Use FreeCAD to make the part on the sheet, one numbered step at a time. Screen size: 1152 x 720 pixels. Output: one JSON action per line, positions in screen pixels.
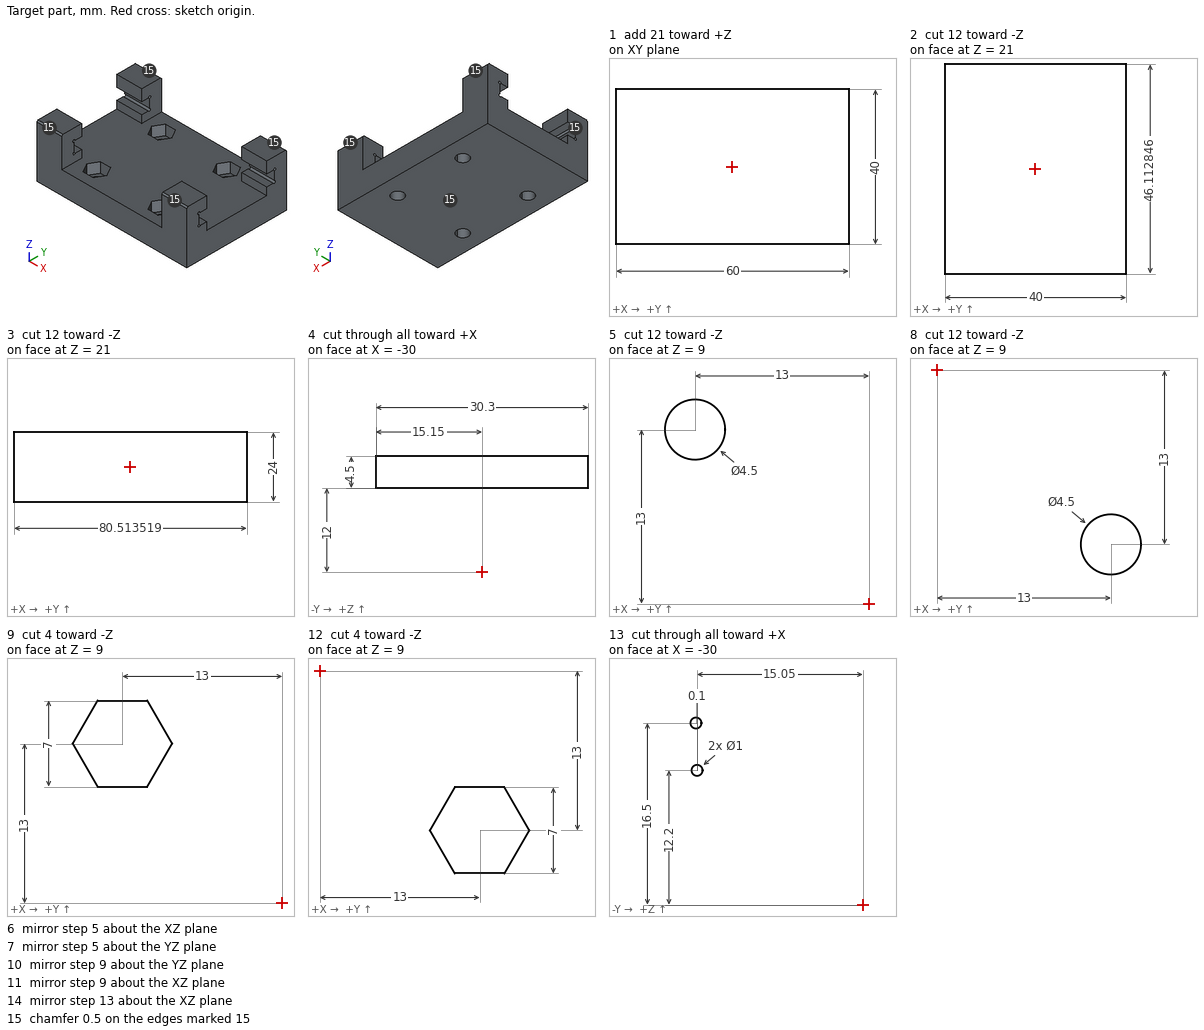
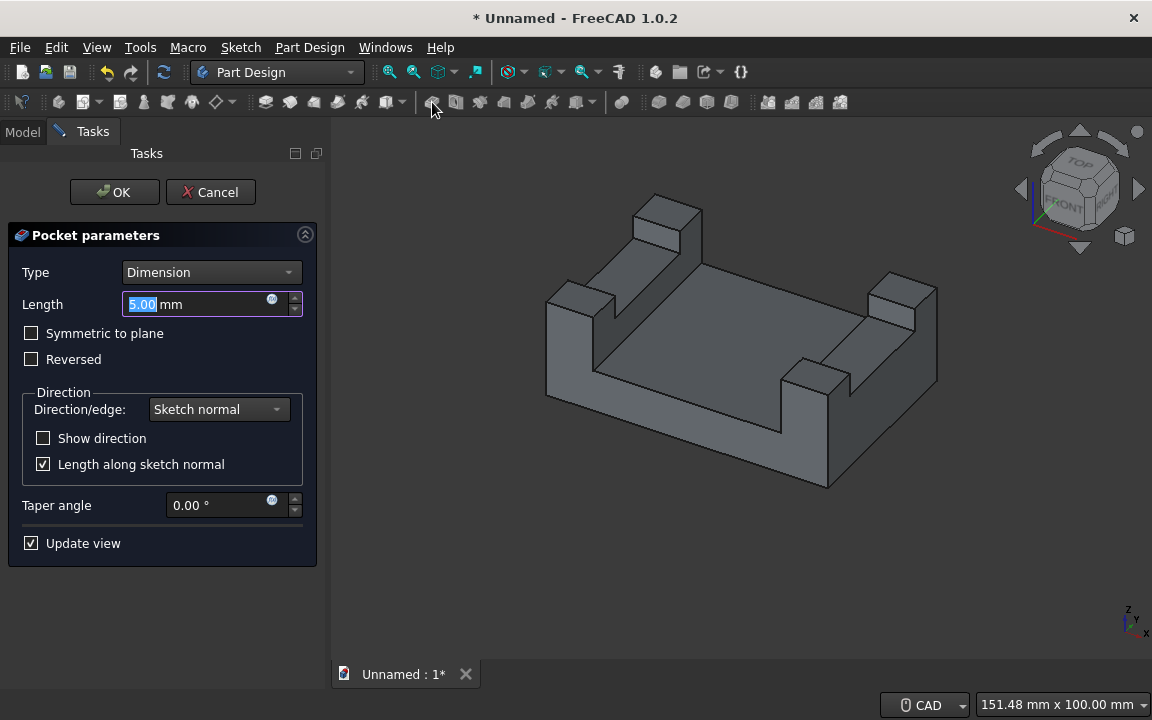
{"action": "type", "text": "12"}
{"action": "key", "text": "Tab"}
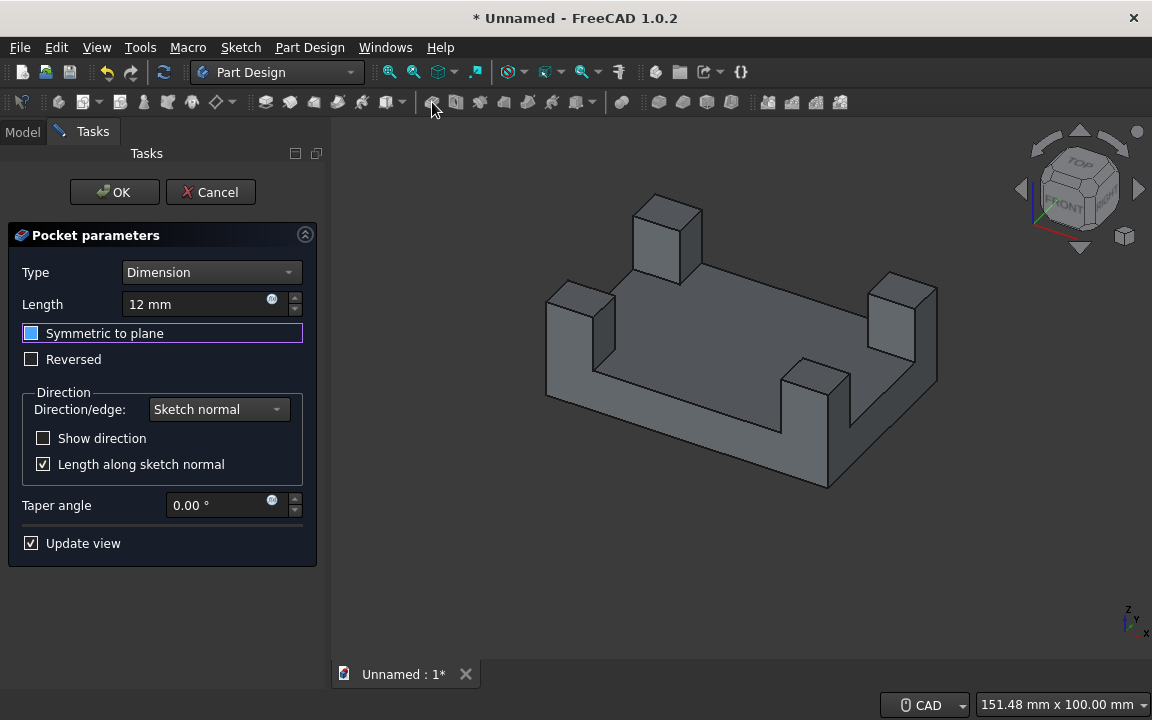
{"action": "left_click", "coordinate": [115, 192]}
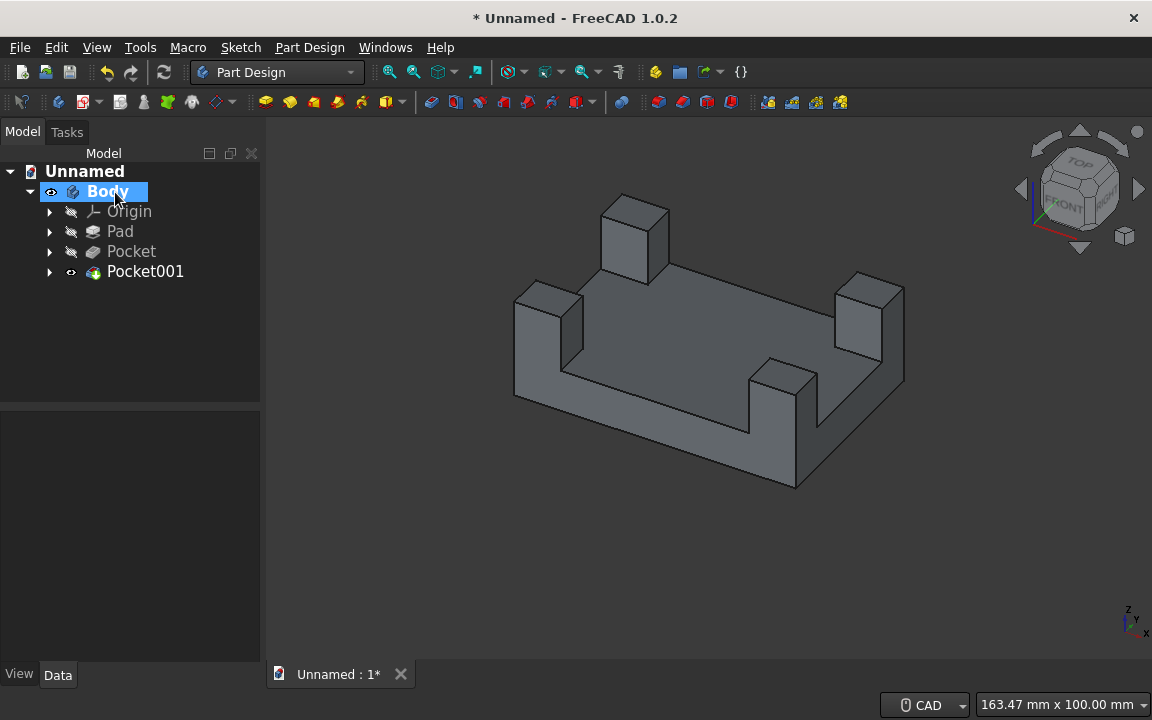
{"action": "key", "text": "6"}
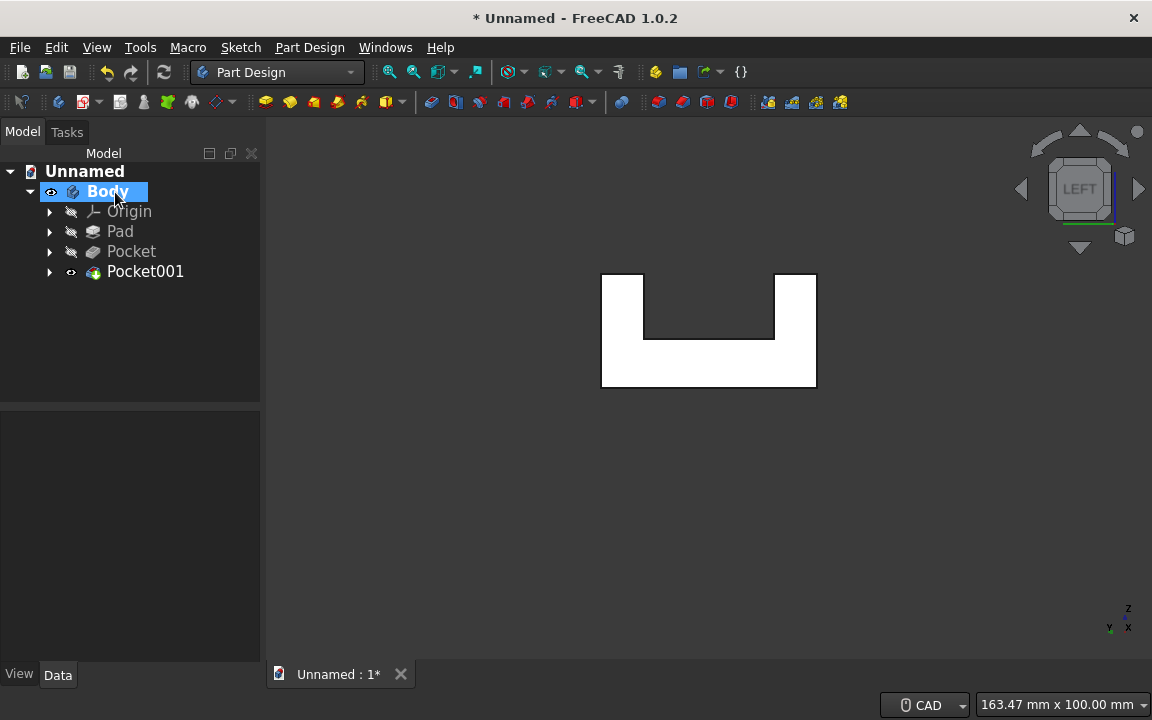
{"action": "left_click", "coordinate": [390, 72]}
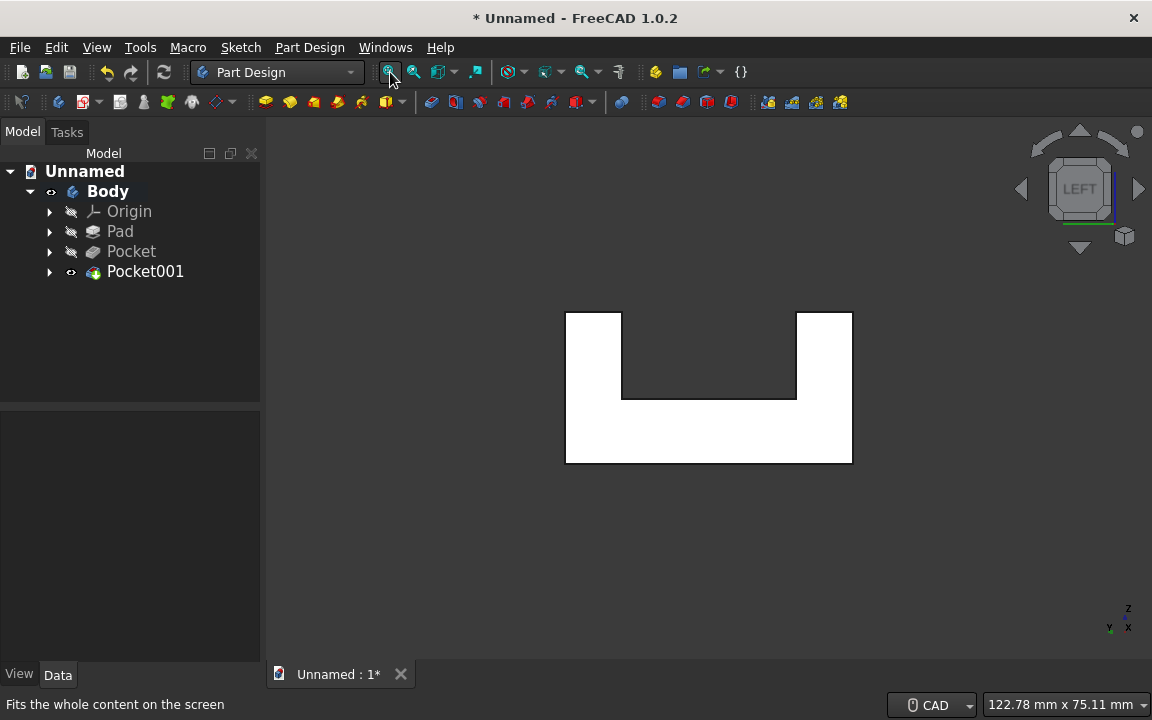
{"action": "left_click", "coordinate": [627, 430]}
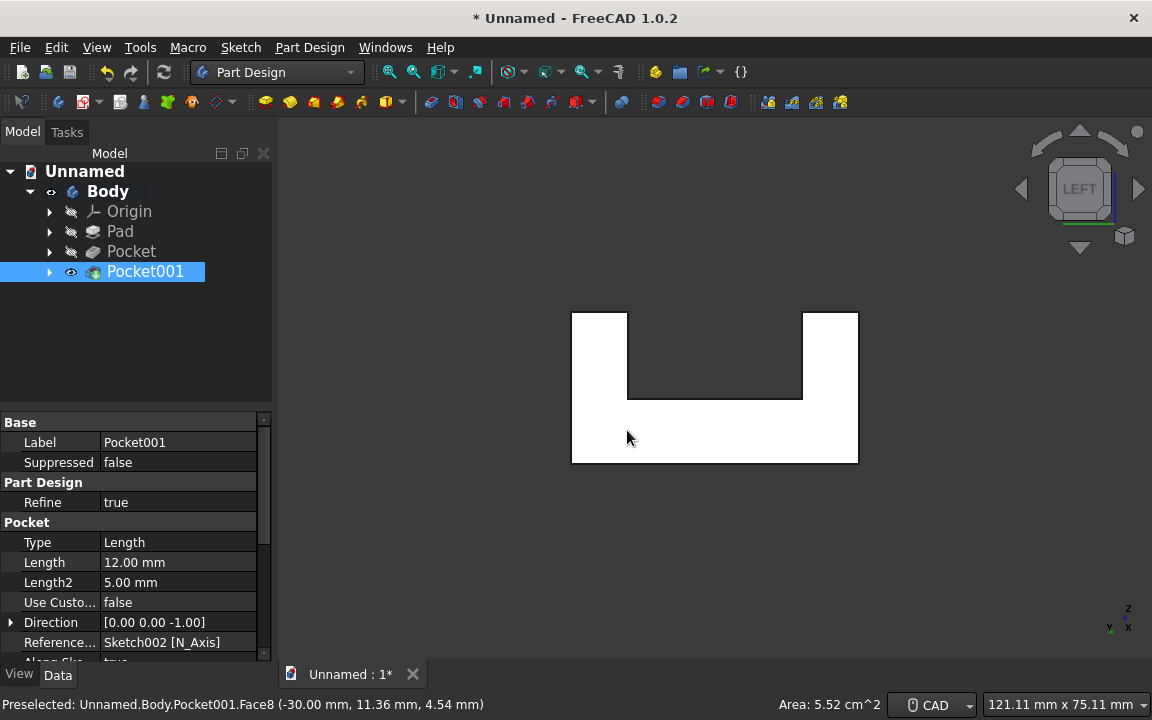
{"action": "left_click", "coordinate": [84, 102]}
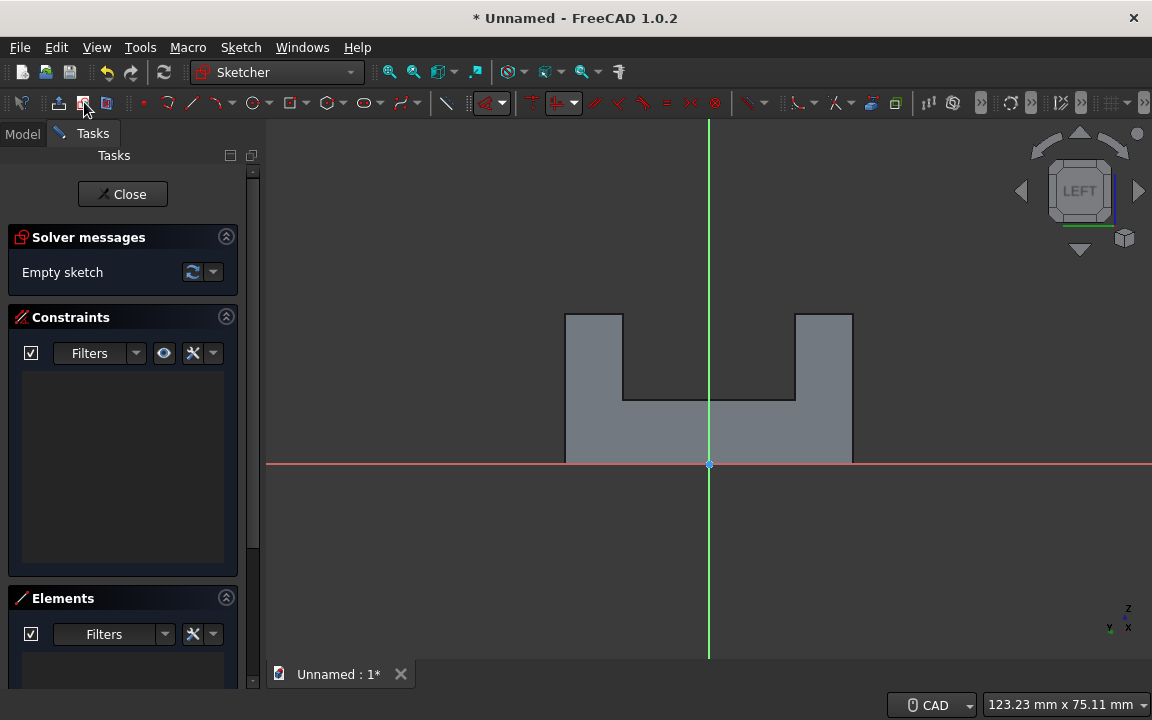
{"action": "scroll", "coordinate": [765, 418], "scroll_direction": "up", "scroll_amount": 4}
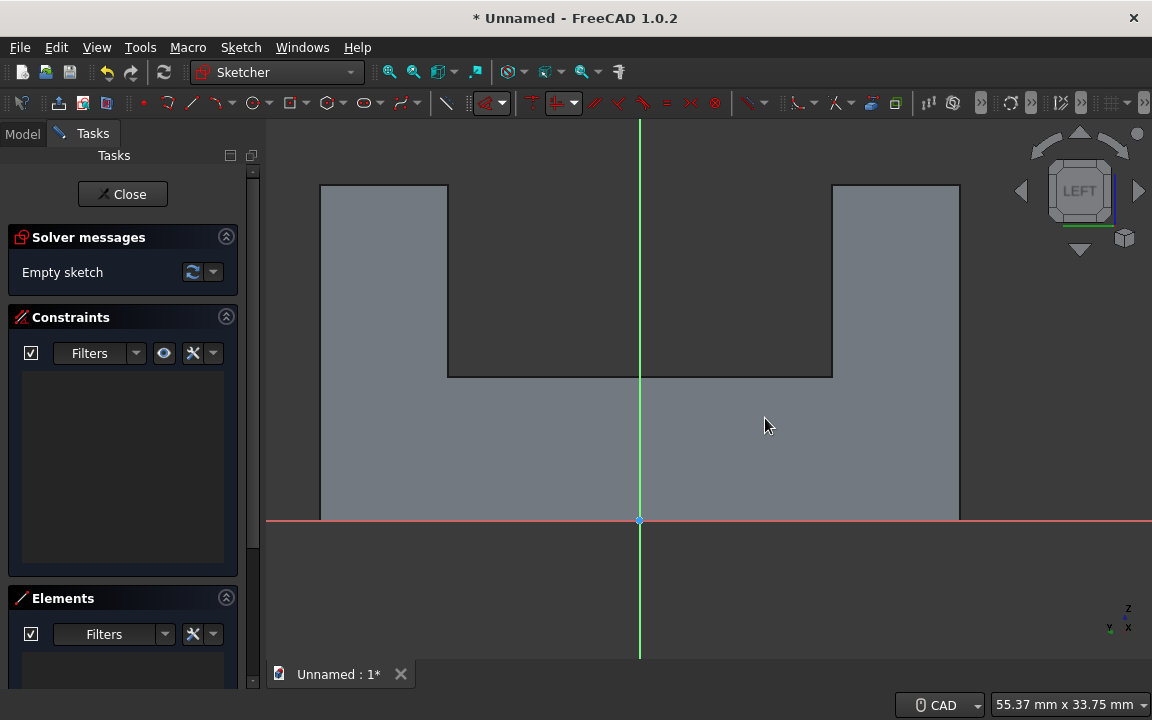
{"action": "left_click", "coordinate": [308, 104]}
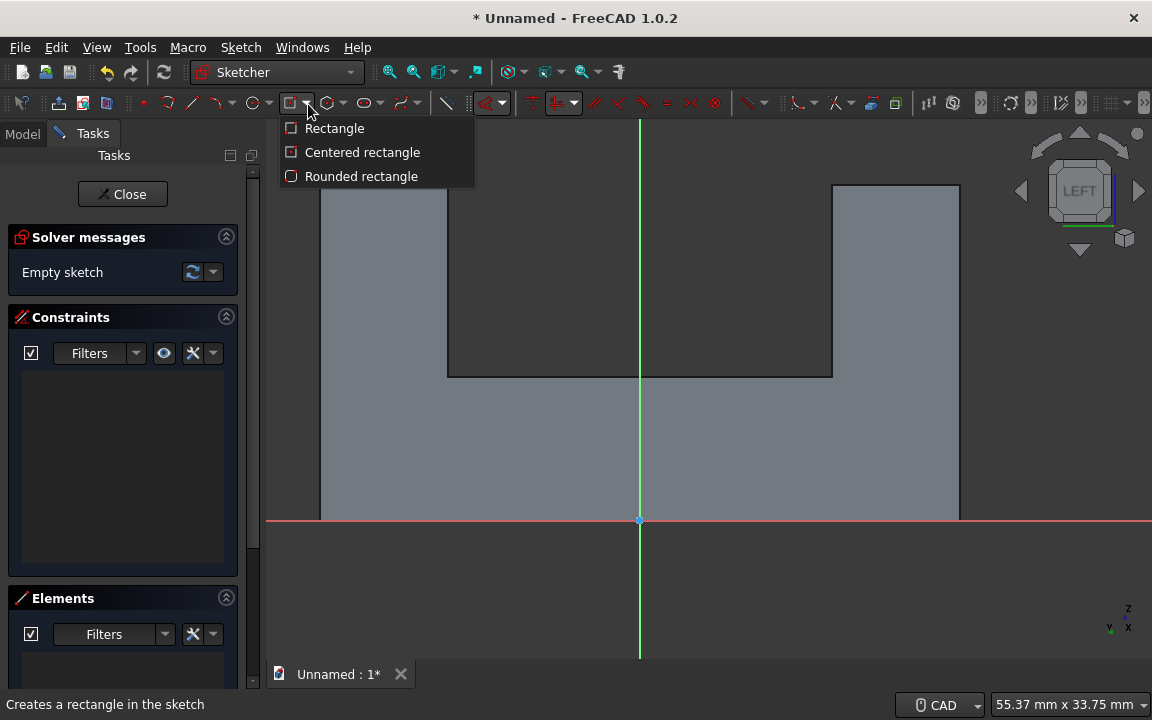
{"action": "left_click", "coordinate": [378, 128]}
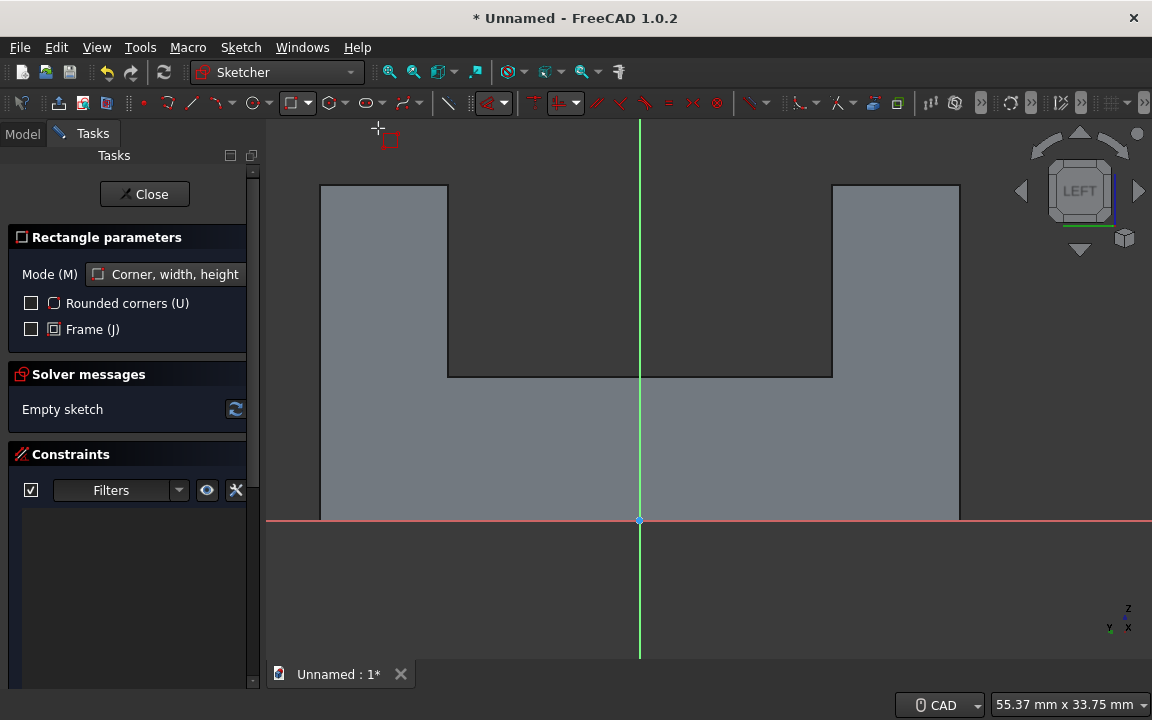
{"action": "left_click", "coordinate": [397, 257]}
{"action": "left_click", "coordinate": [882, 329]}
{"action": "key", "text": "Escape"}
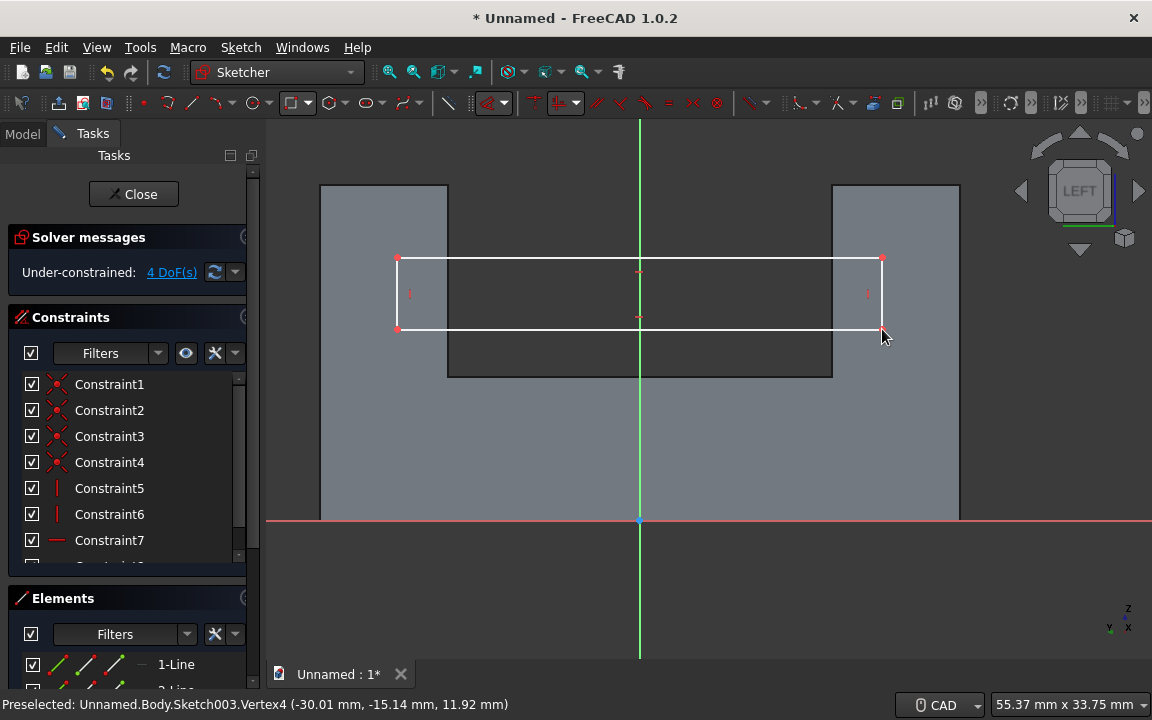
{"action": "left_click", "coordinate": [397, 280]}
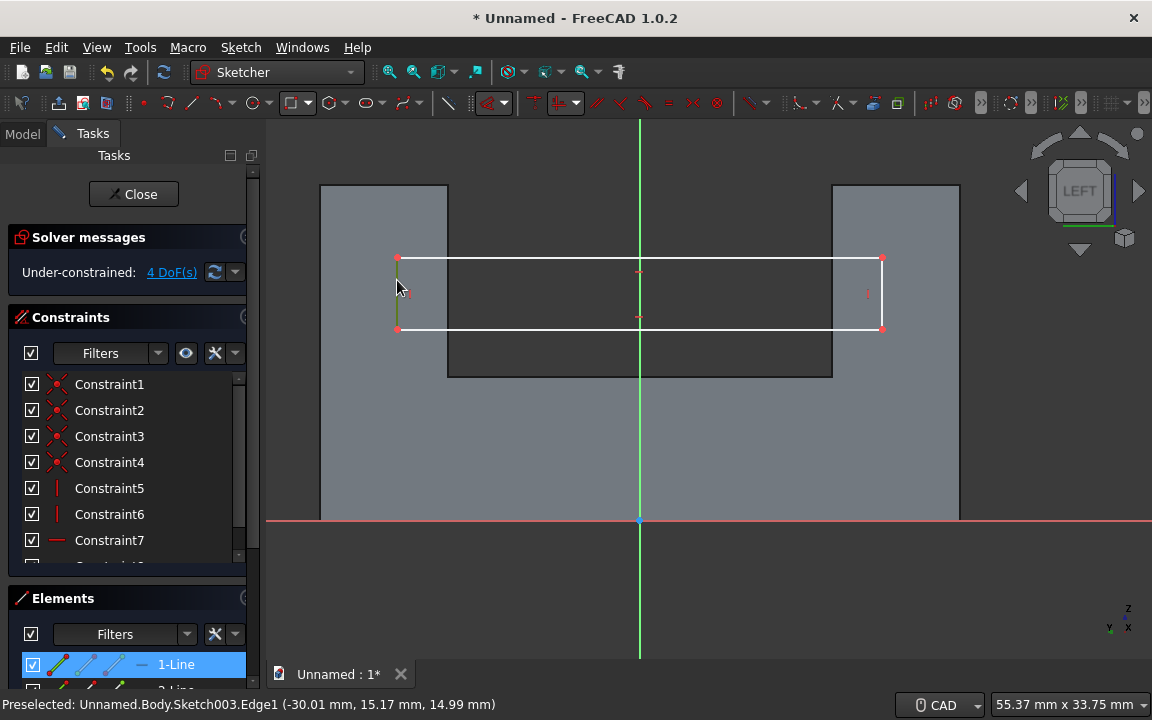
{"action": "left_click", "coordinate": [506, 104]}